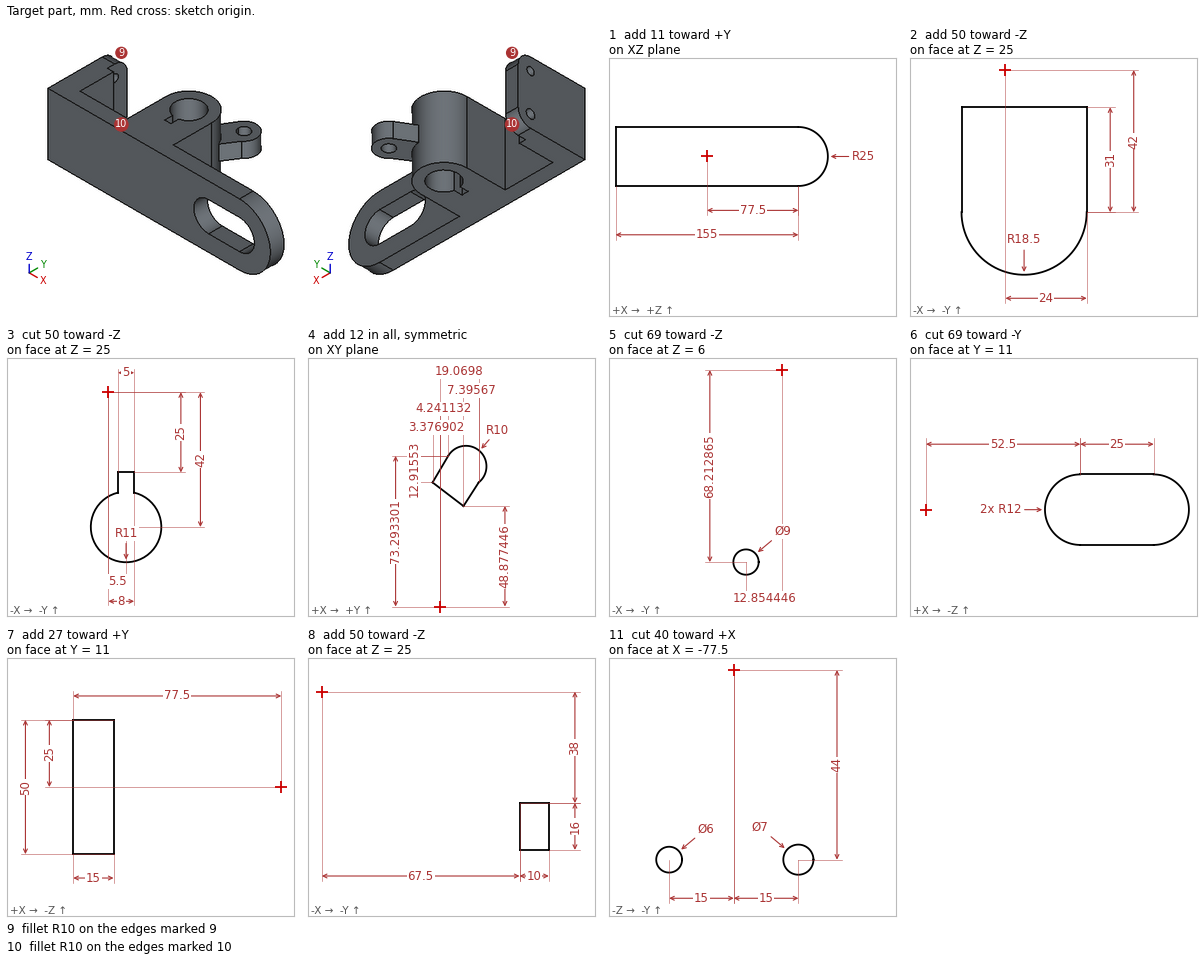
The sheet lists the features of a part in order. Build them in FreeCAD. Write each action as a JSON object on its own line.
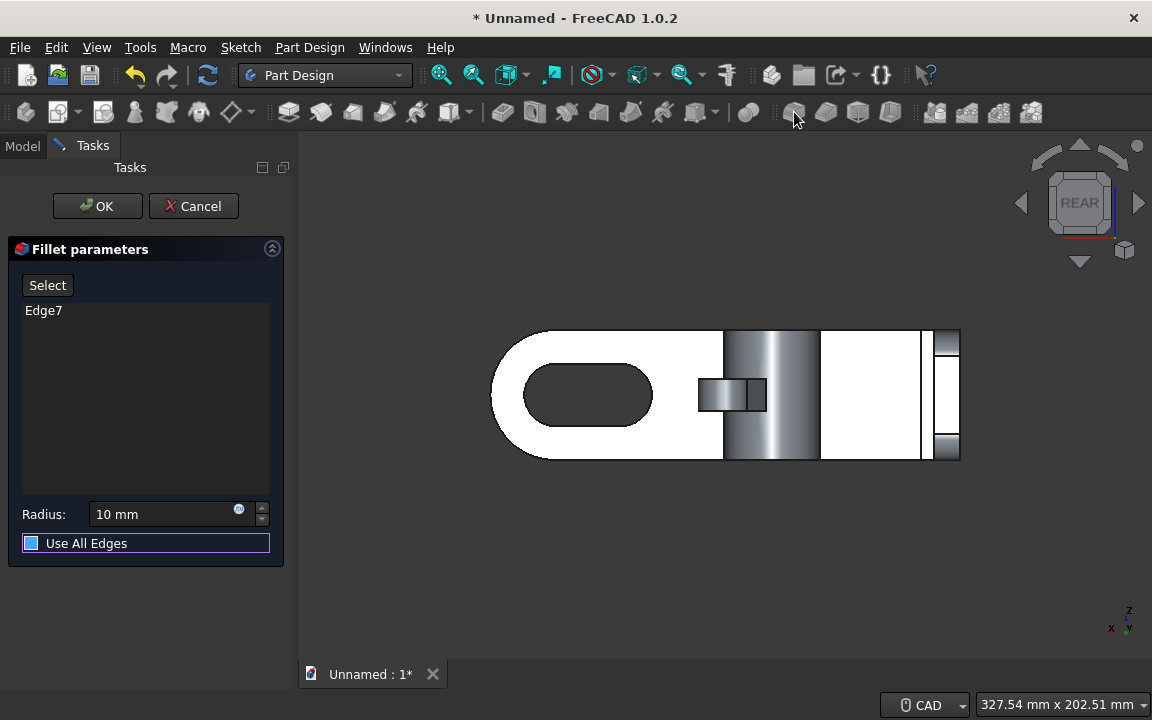
{"action": "left_click", "coordinate": [98, 206]}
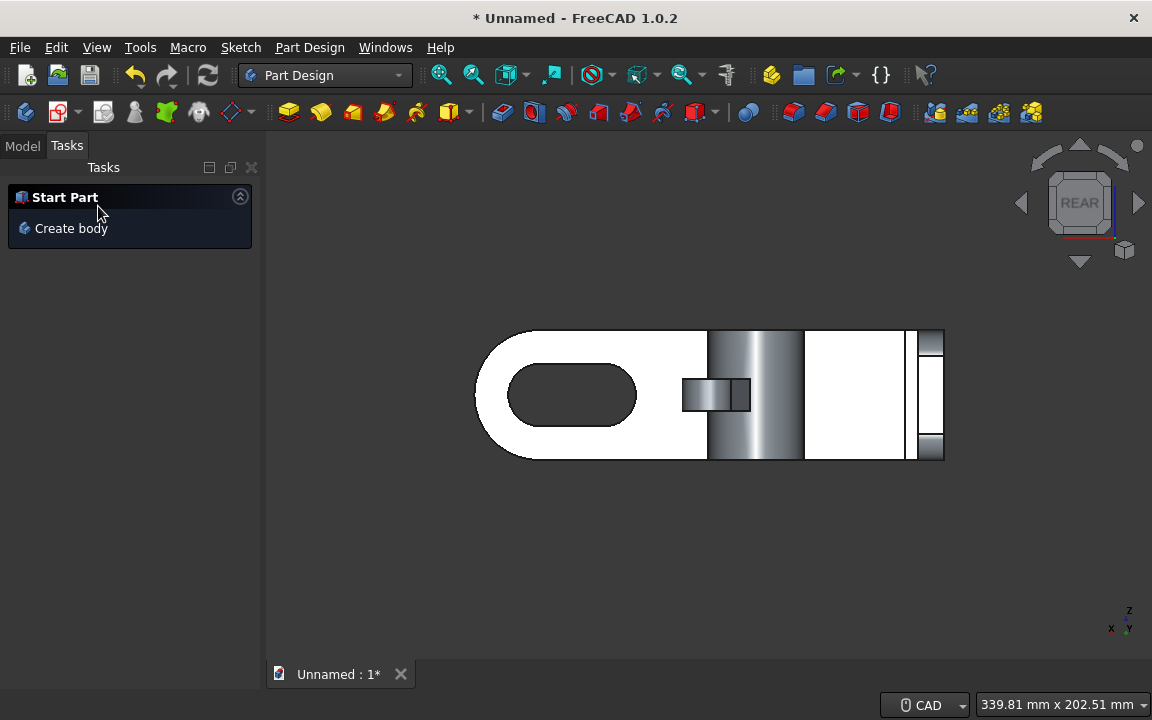
{"action": "key", "text": "6"}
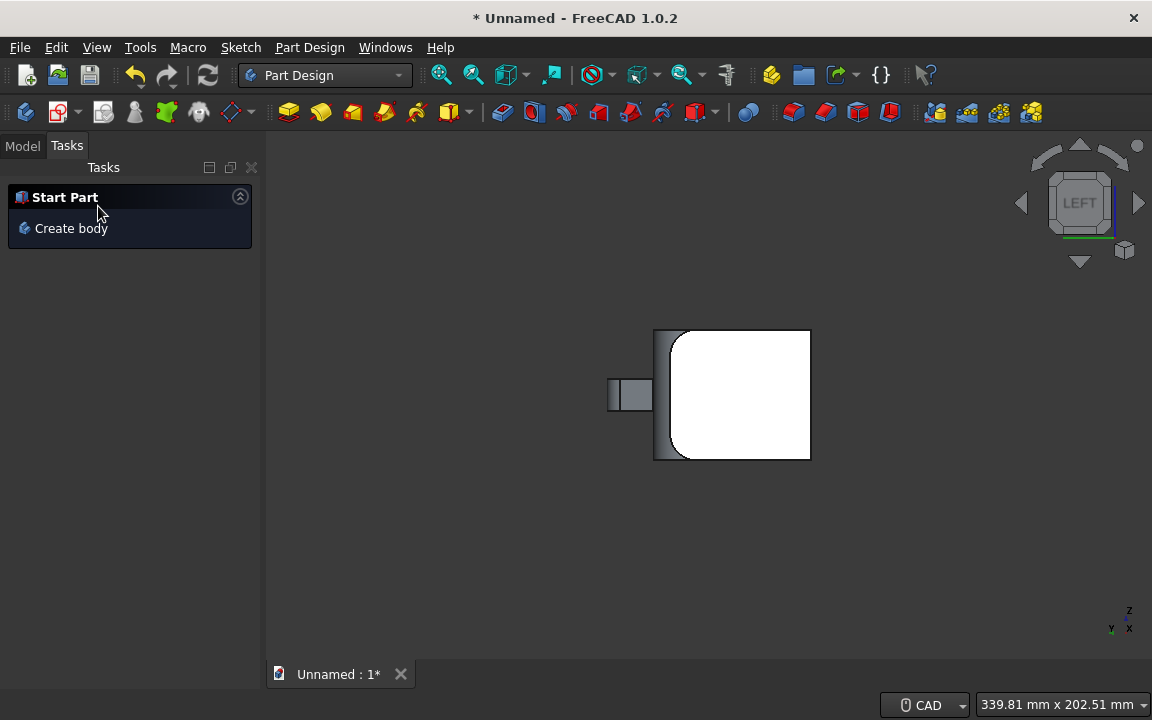
{"action": "left_click", "coordinate": [442, 76]}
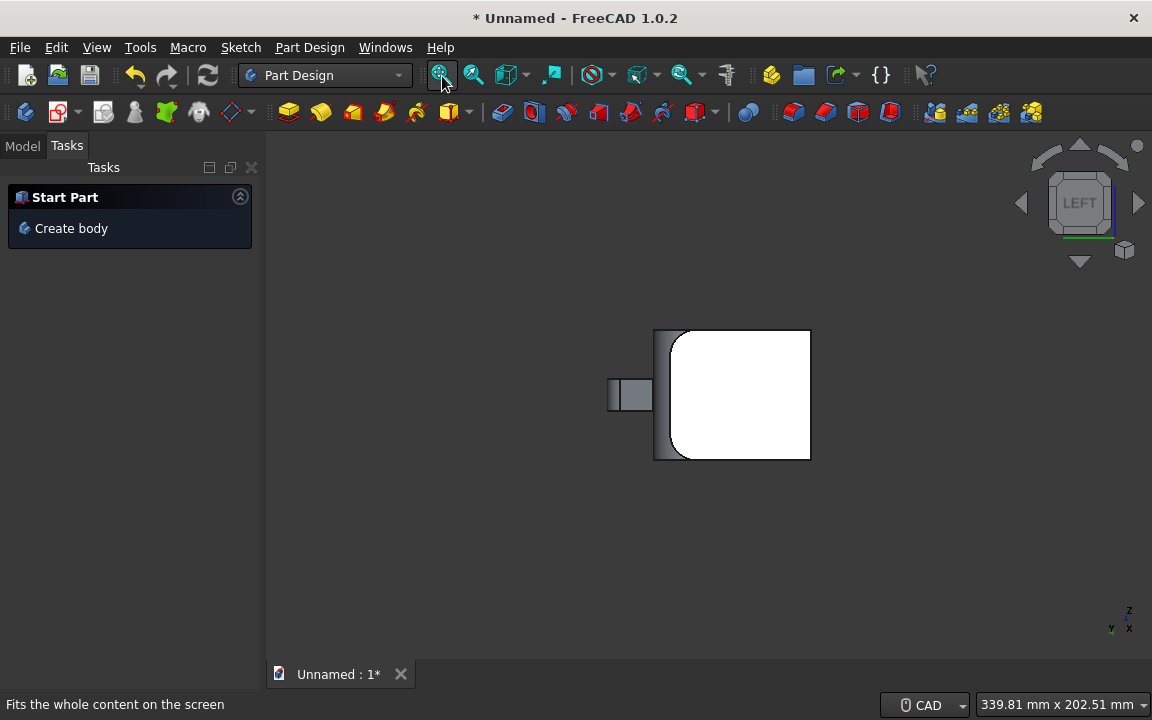
{"action": "left_click", "coordinate": [740, 394]}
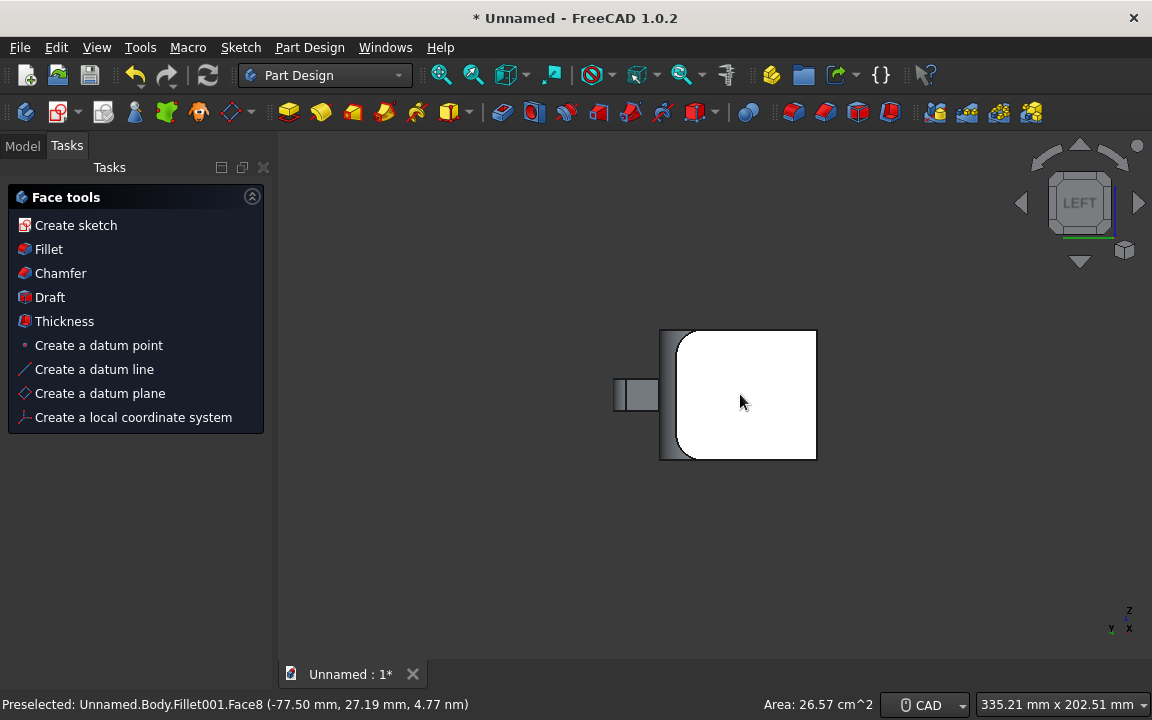
{"action": "left_click", "coordinate": [58, 112]}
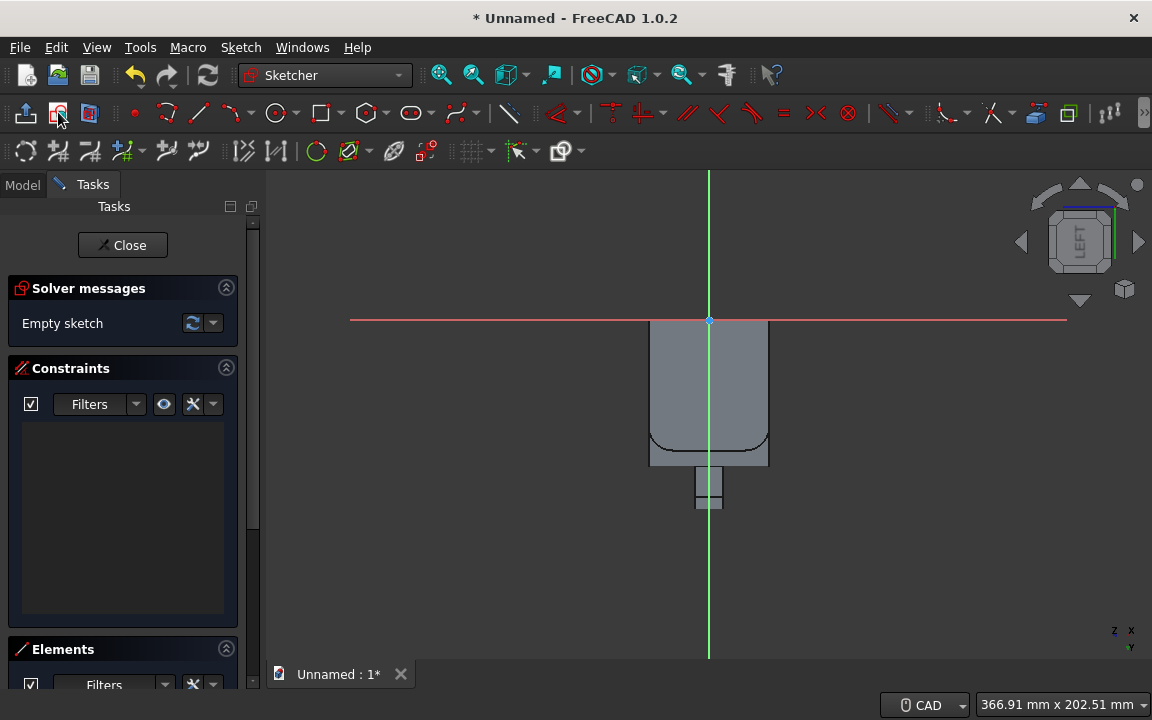
{"action": "scroll", "coordinate": [750, 356], "scroll_direction": "up", "scroll_amount": 5}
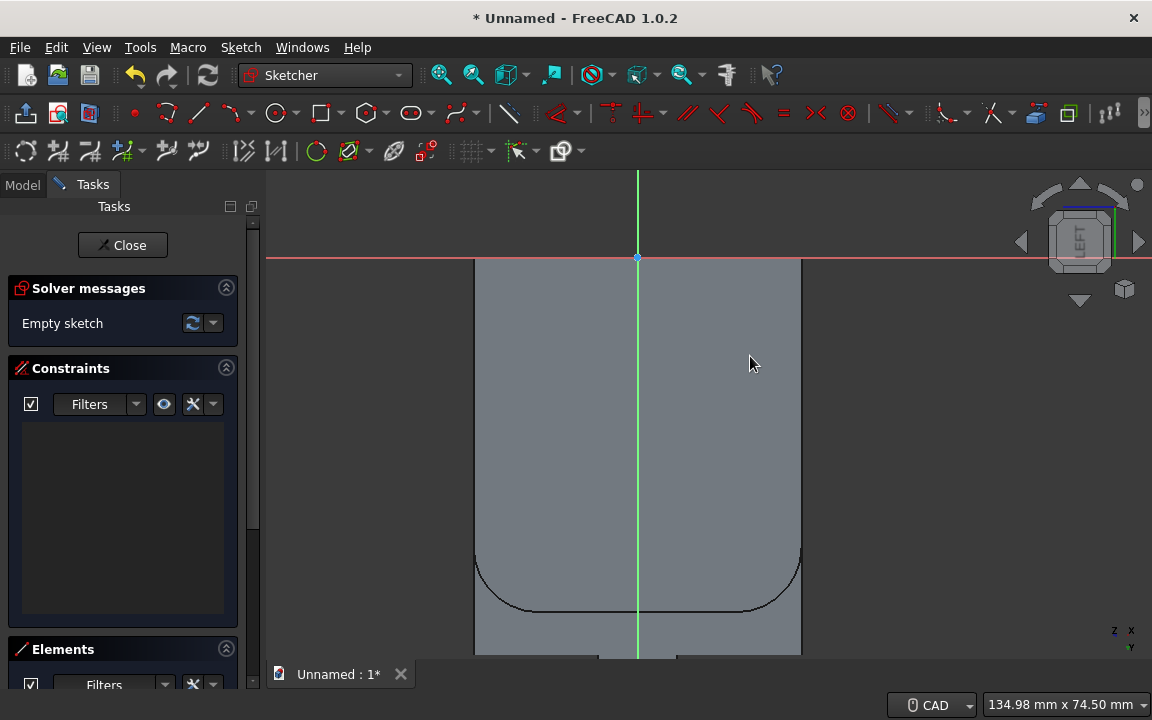
{"action": "left_click", "coordinate": [276, 114]}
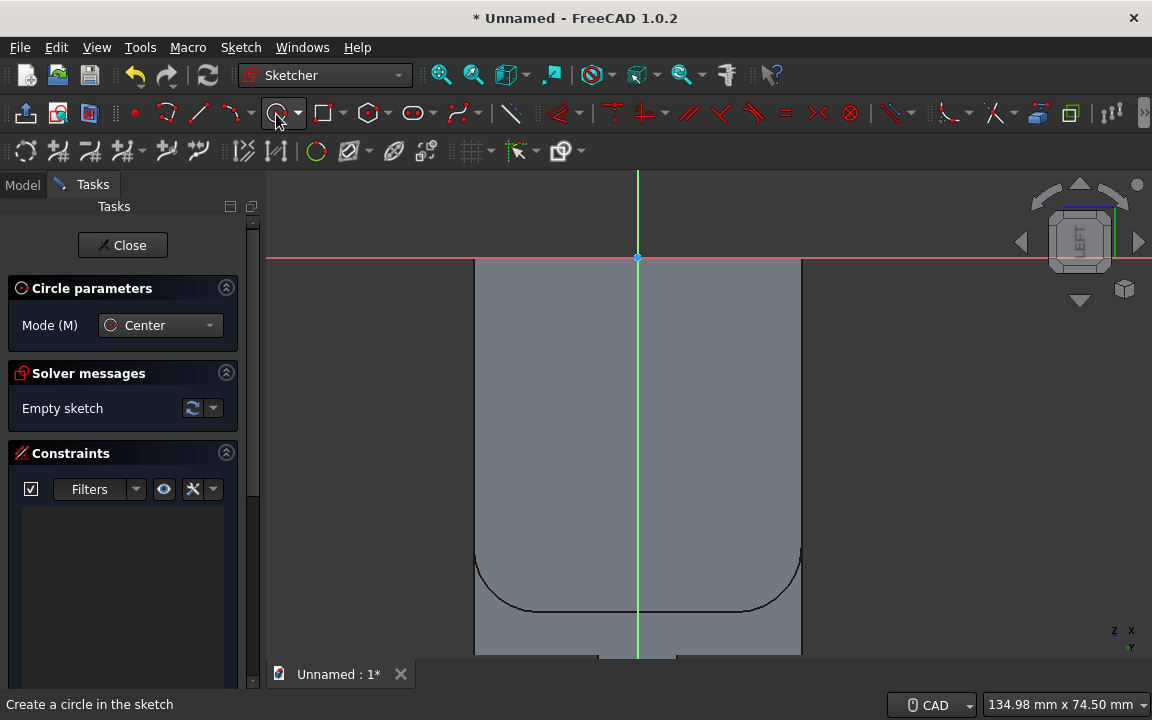
{"action": "left_click", "coordinate": [736, 547]}
{"action": "mouse_move", "coordinate": [752, 530]}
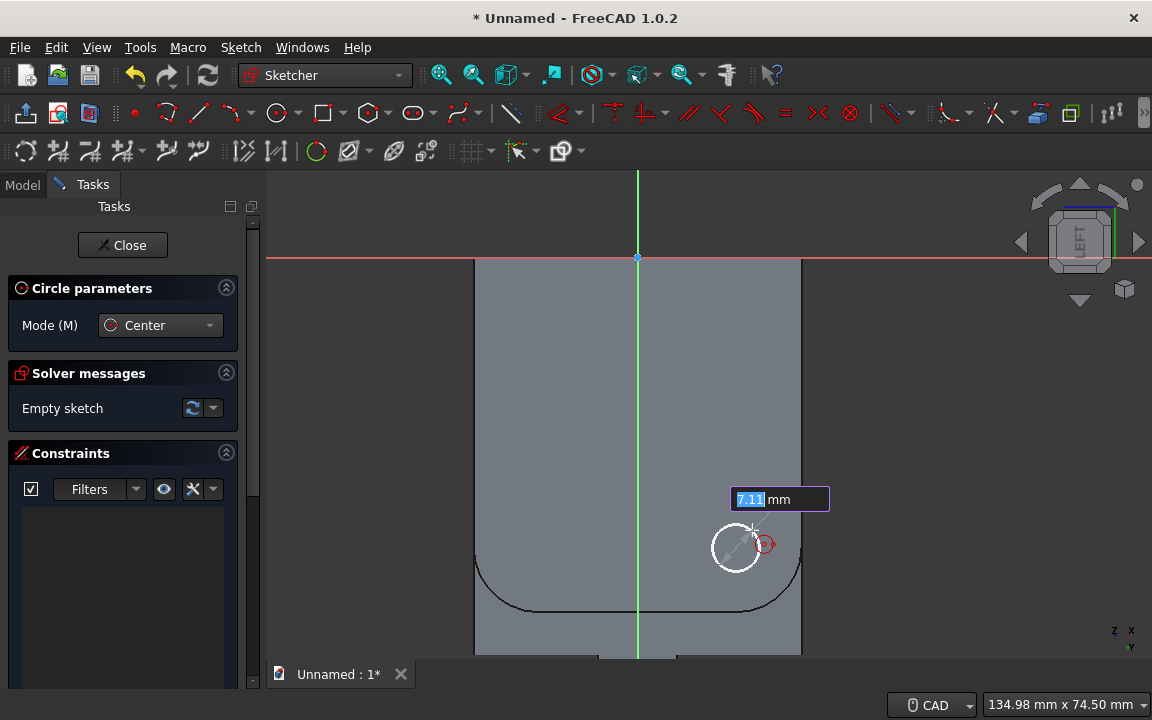
{"action": "type", "text": "7"}
{"action": "key", "text": "Return"}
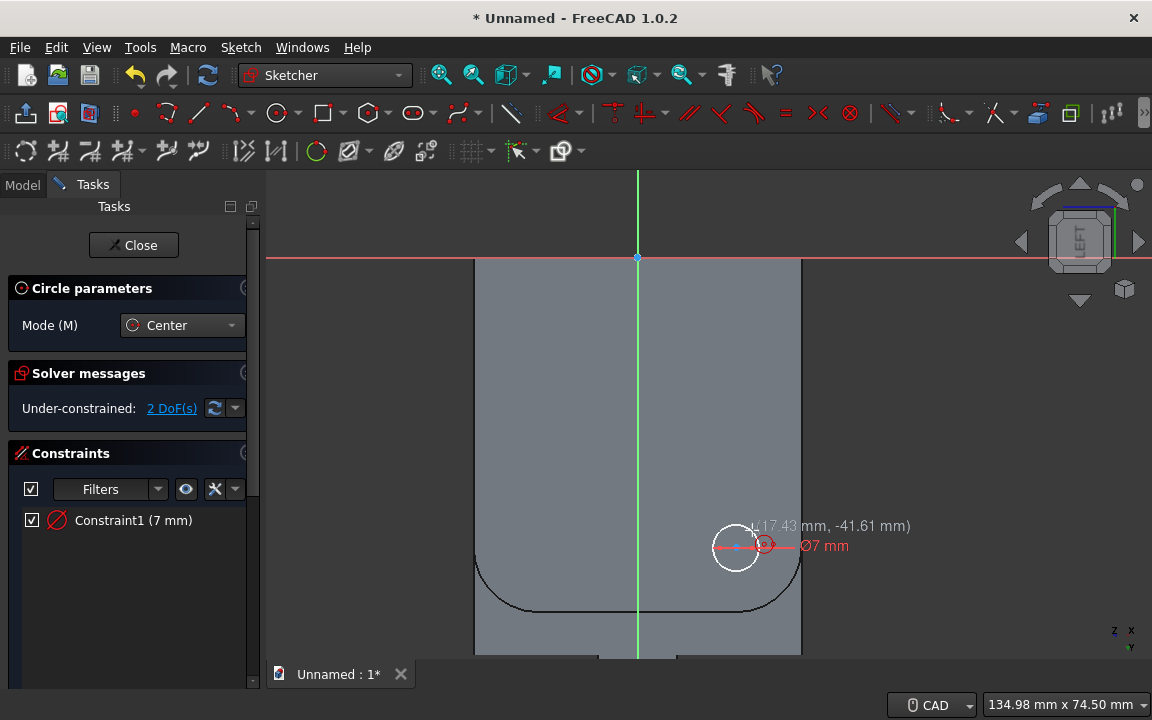
{"action": "left_click", "coordinate": [539, 547]}
{"action": "mouse_move", "coordinate": [553, 533]}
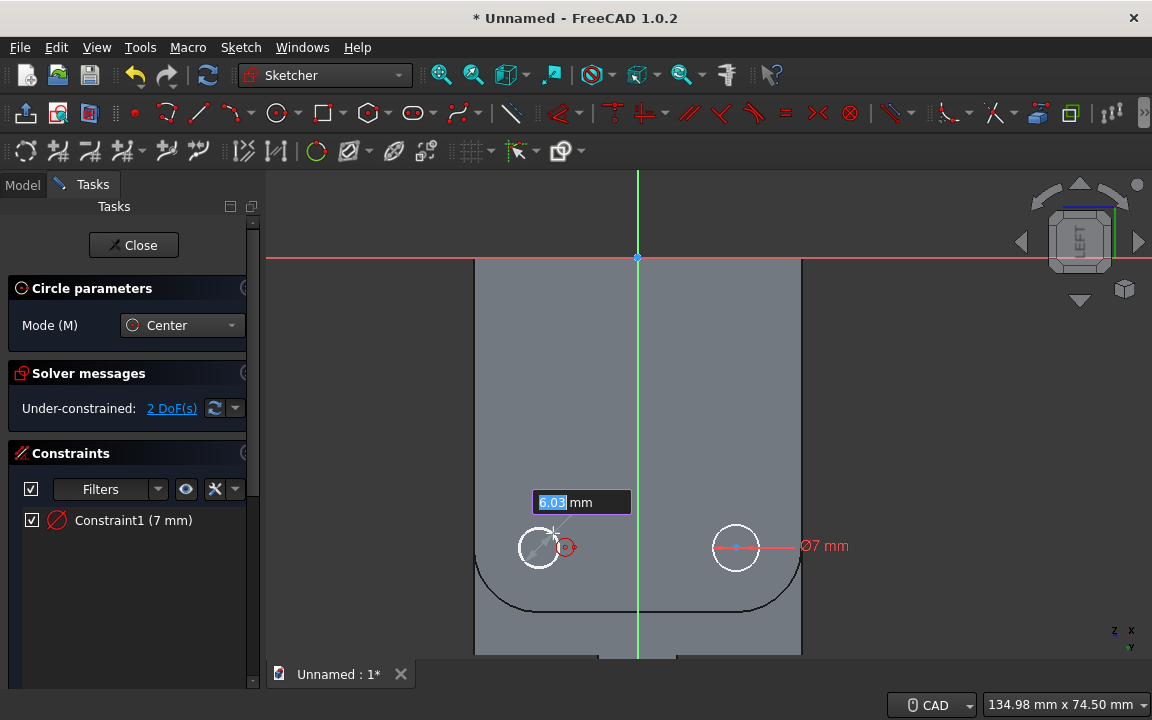
{"action": "type", "text": "6"}
{"action": "key", "text": "Return"}
{"action": "key", "text": "Escape"}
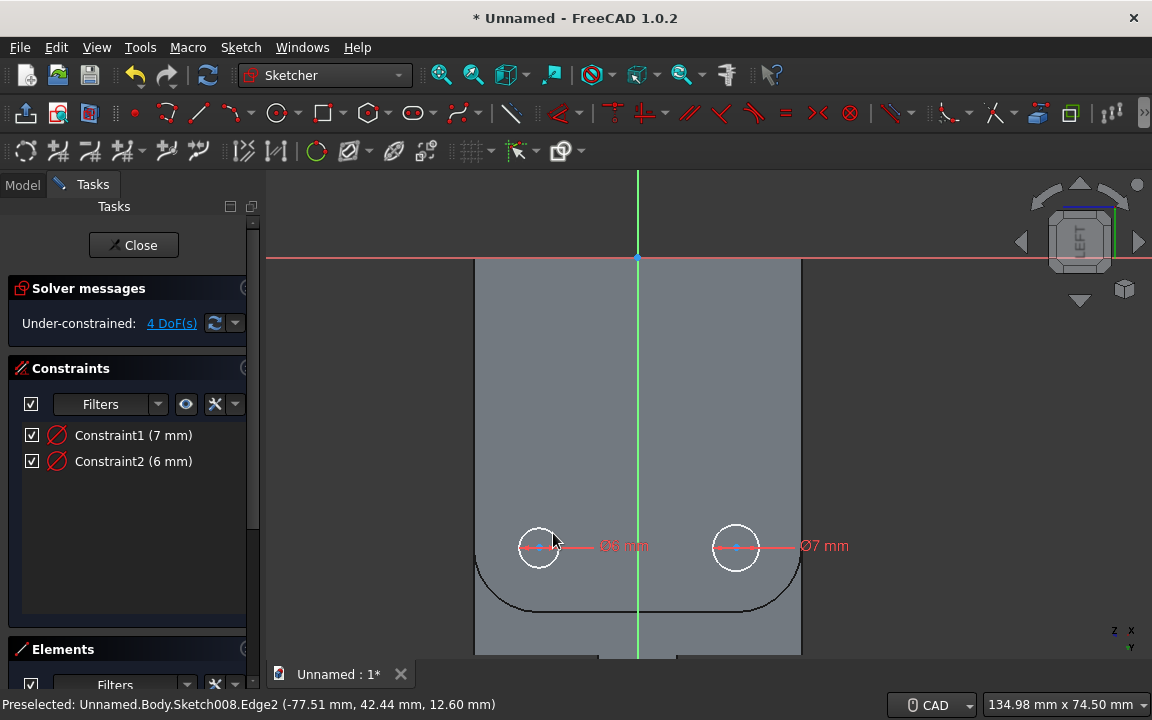
{"action": "left_click", "coordinate": [736, 548]}